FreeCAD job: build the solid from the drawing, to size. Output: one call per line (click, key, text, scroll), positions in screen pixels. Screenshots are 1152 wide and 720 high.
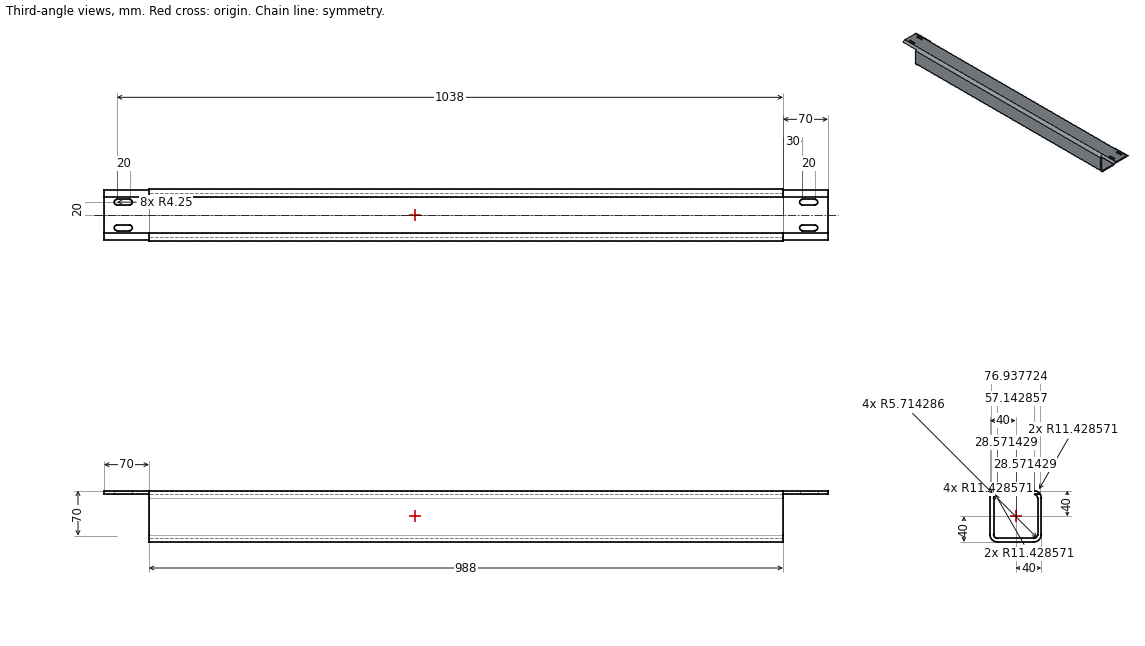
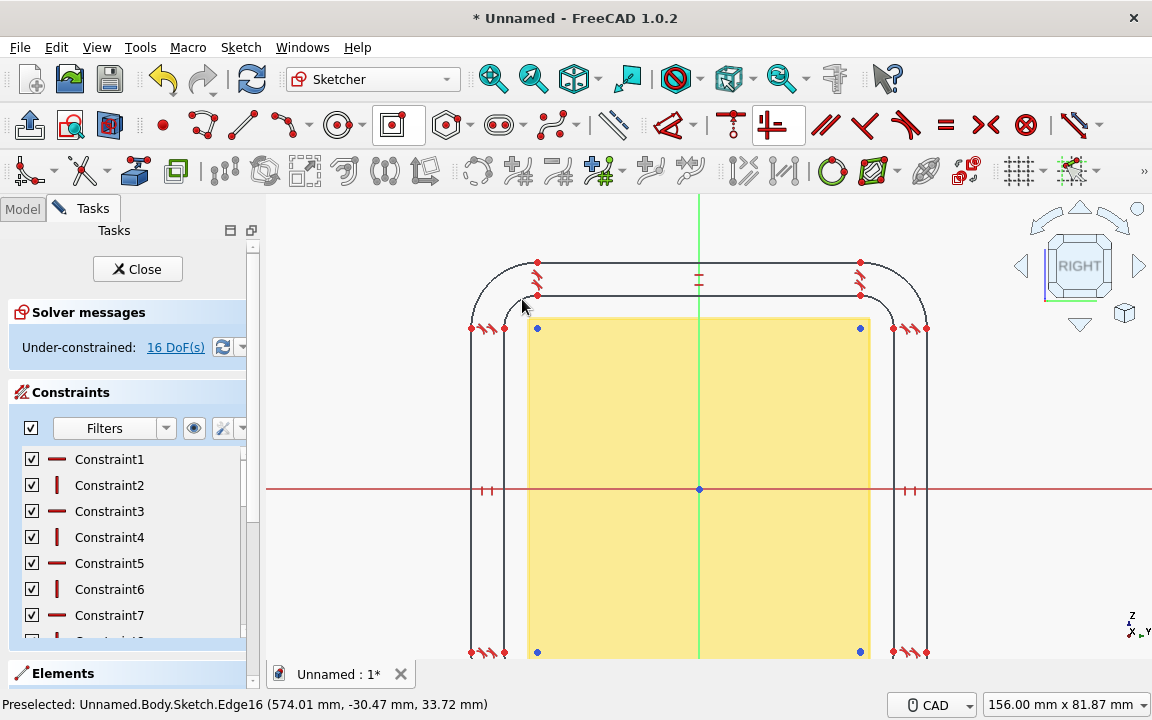
click(920, 299)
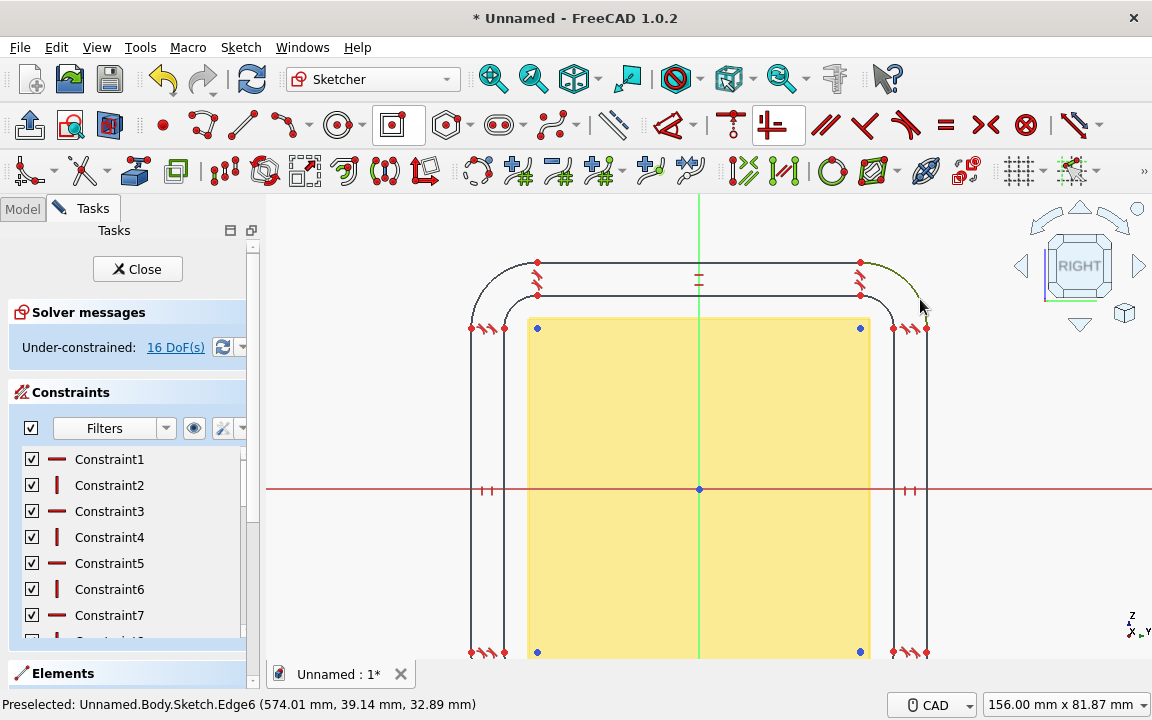
click(890, 314)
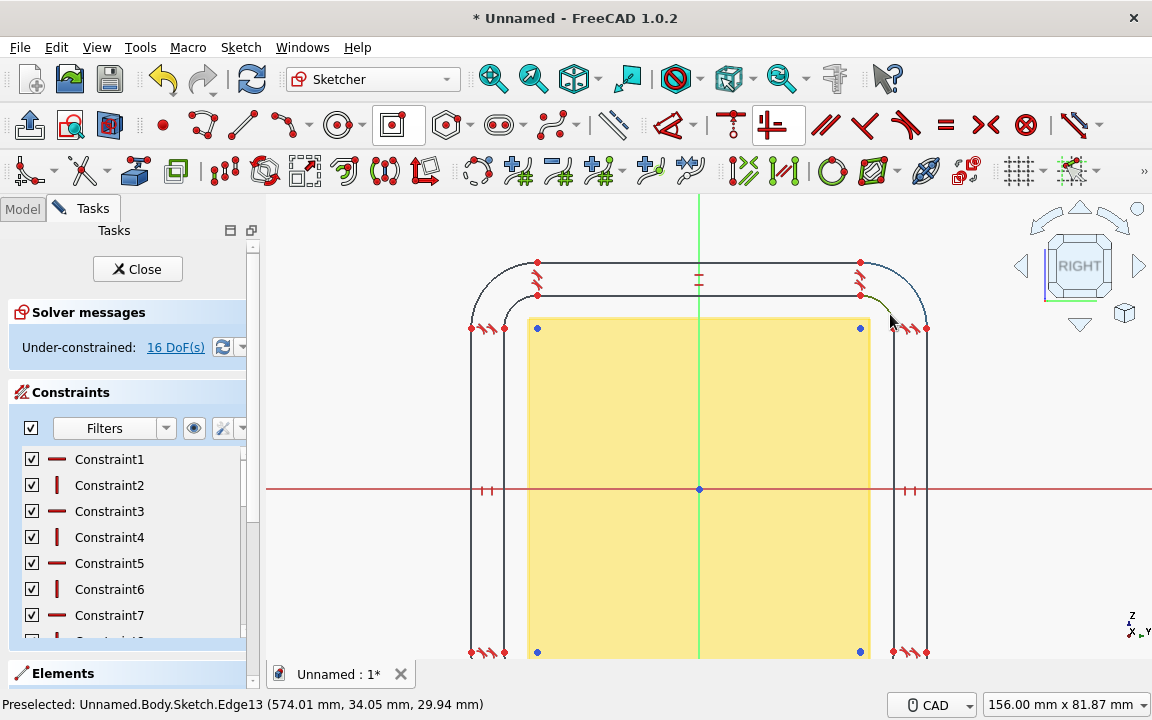
key(c)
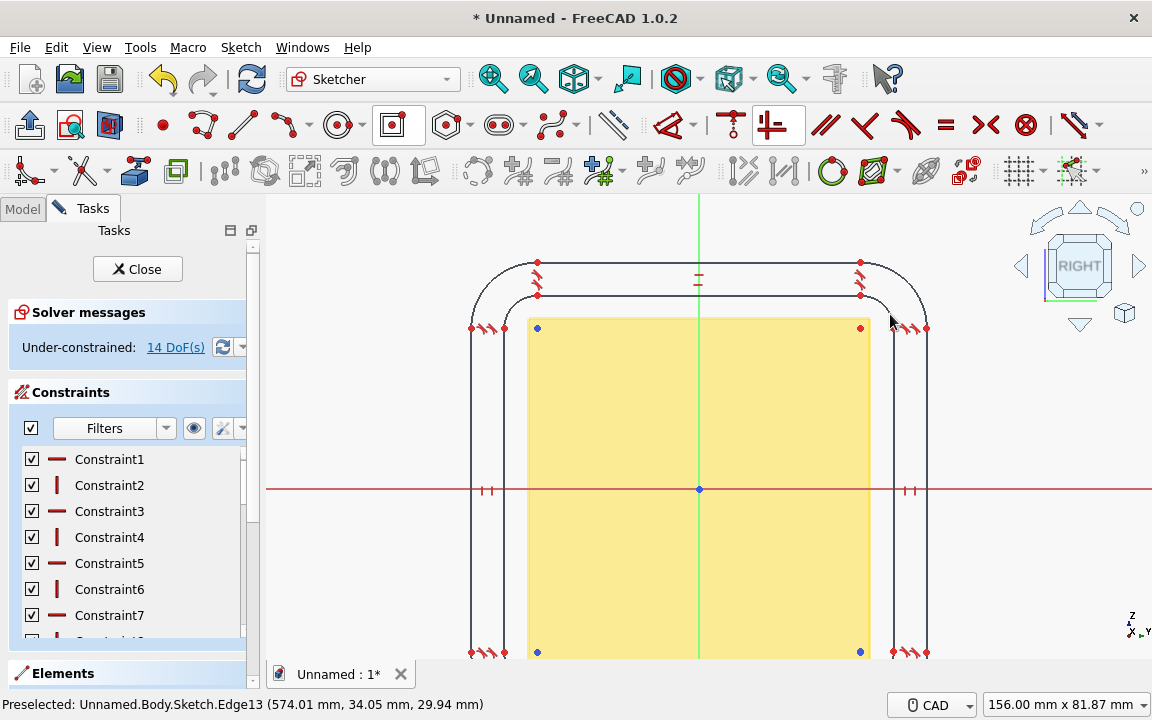
scroll(521, 299, down, 2)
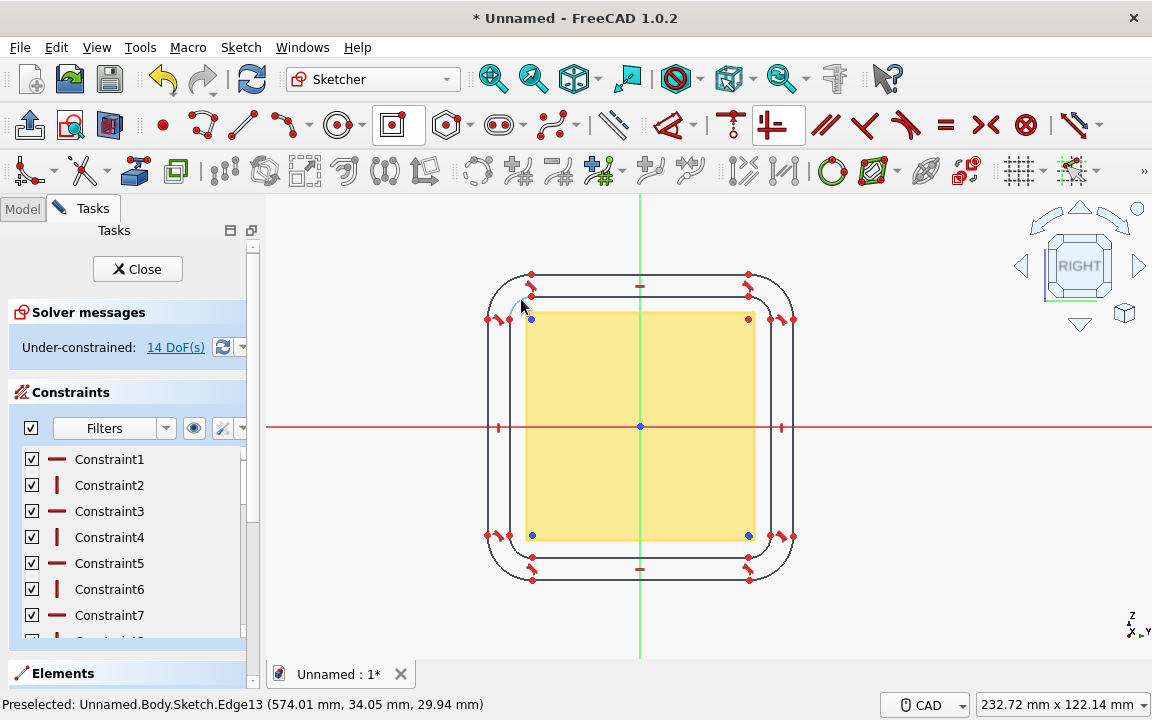
click(769, 575)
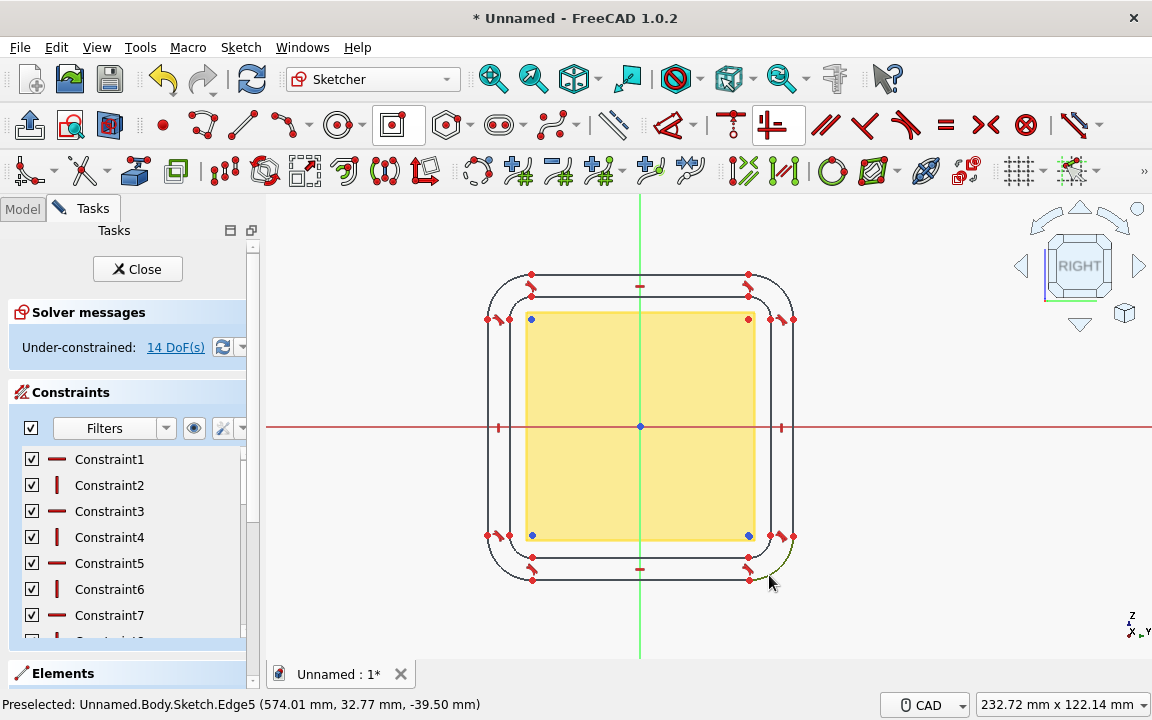
scroll(759, 556, up, 2)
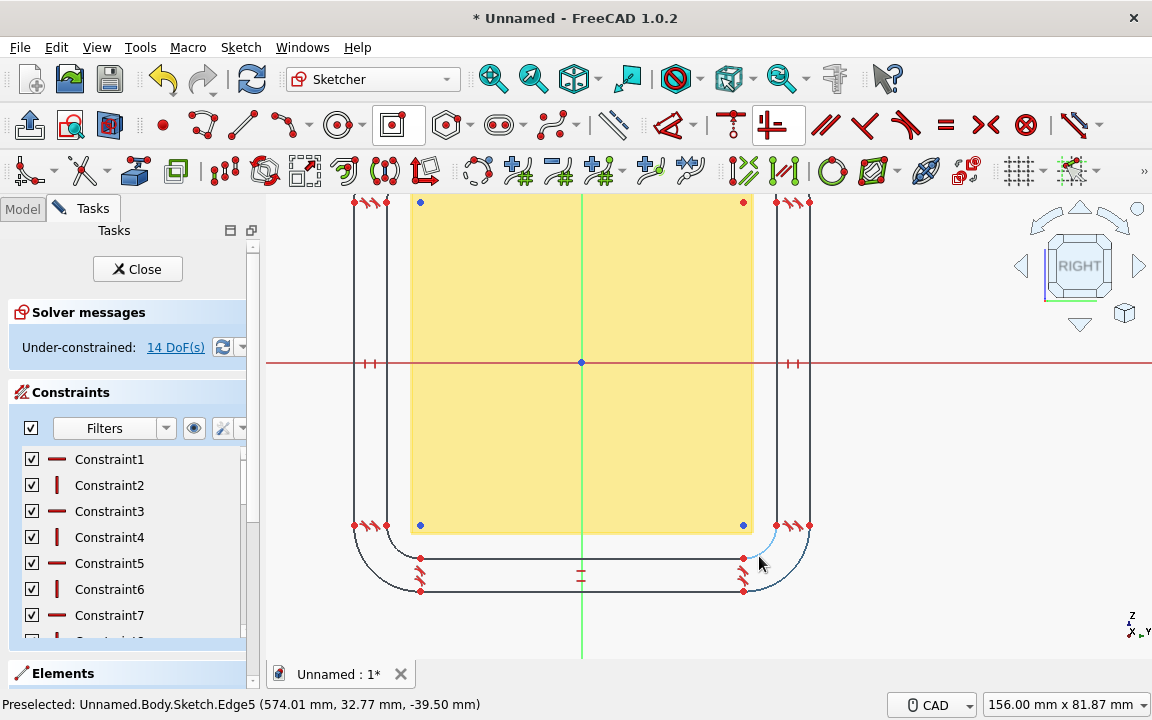
click(758, 555)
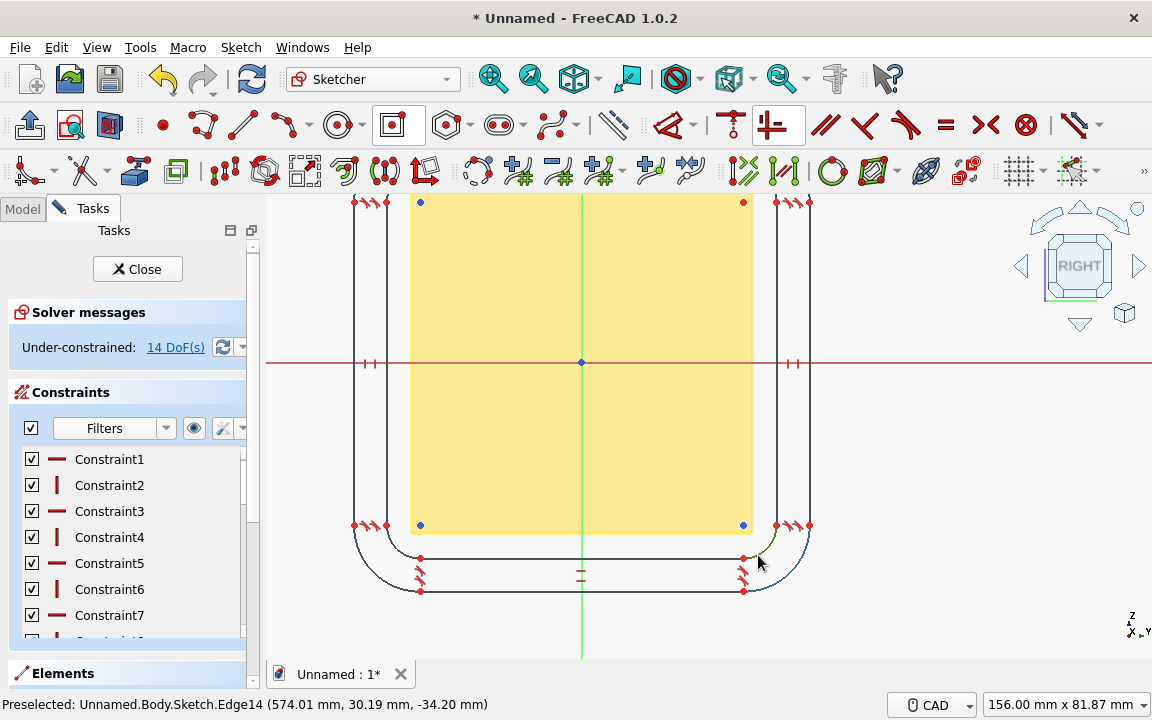
click(732, 126)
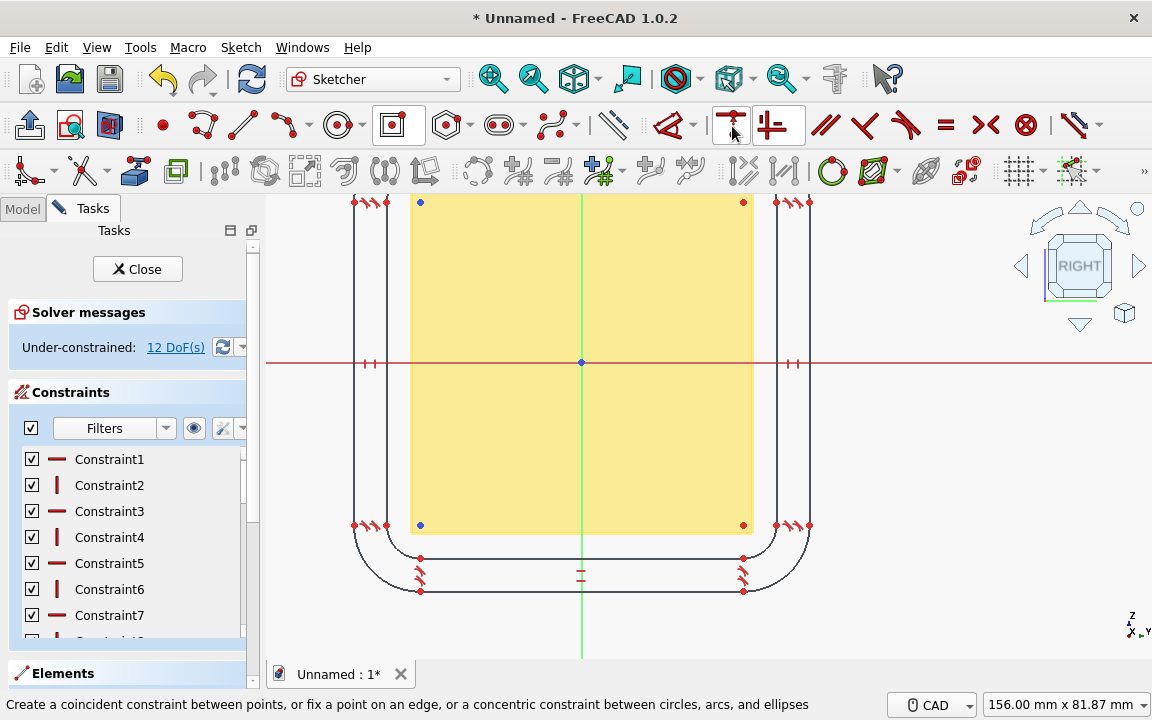
click(361, 556)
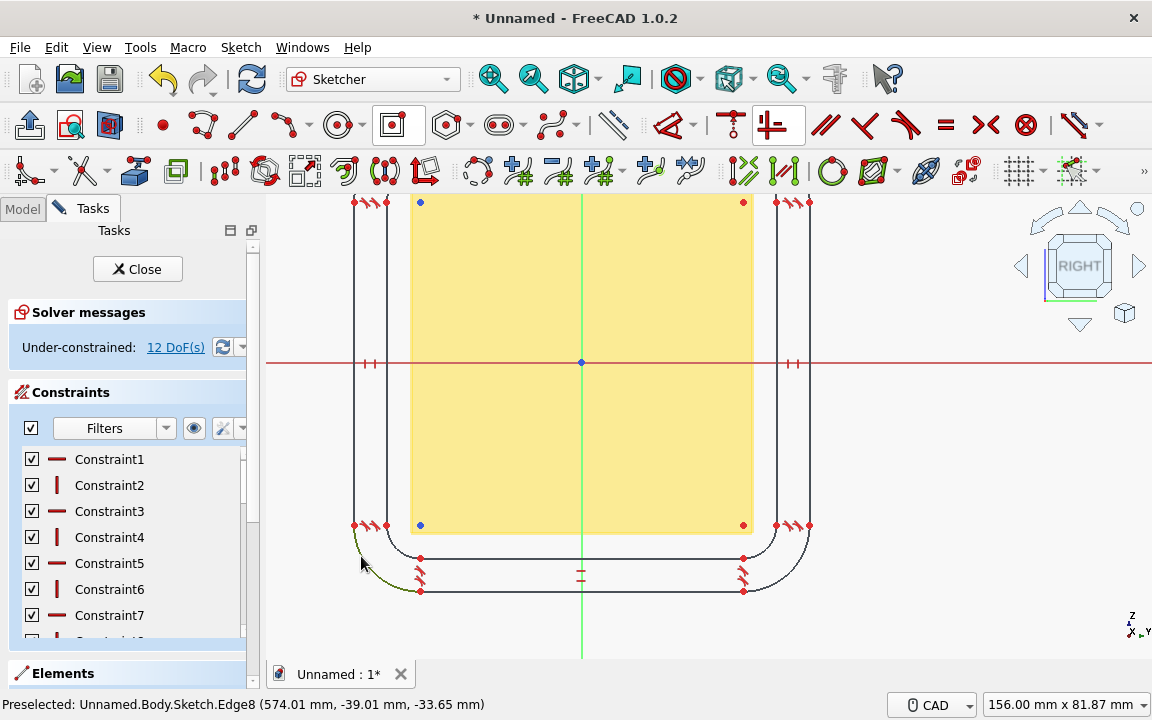
click(391, 540)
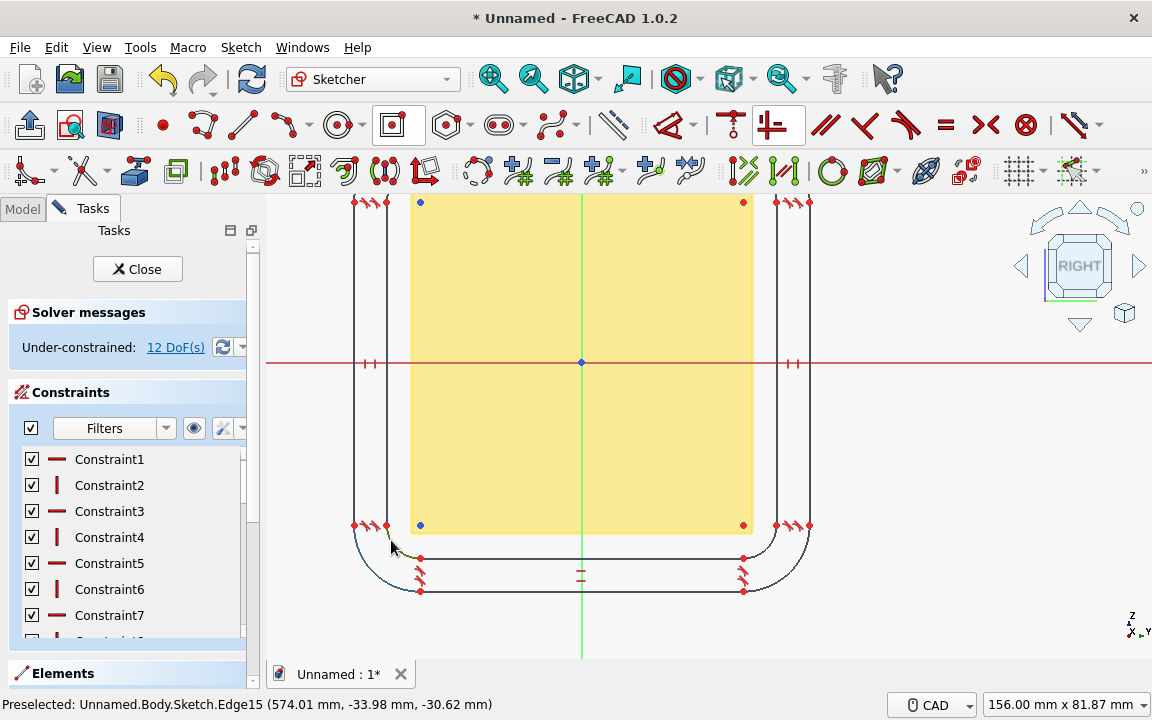
click(732, 126)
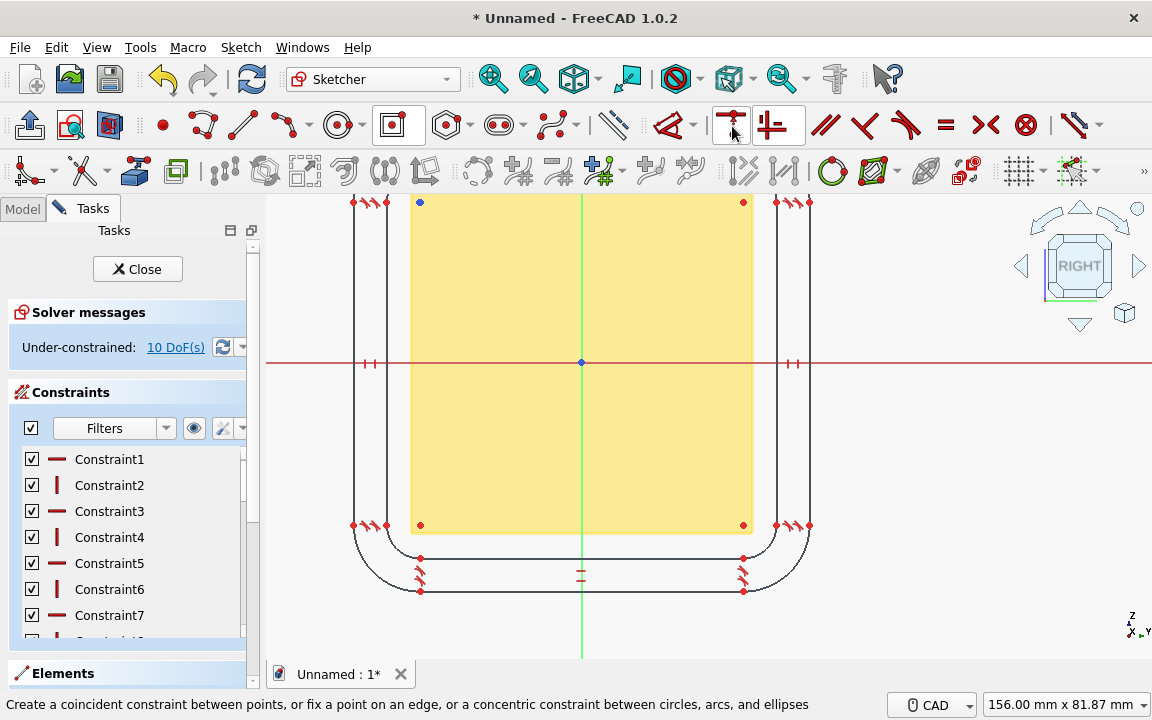
click(773, 584)